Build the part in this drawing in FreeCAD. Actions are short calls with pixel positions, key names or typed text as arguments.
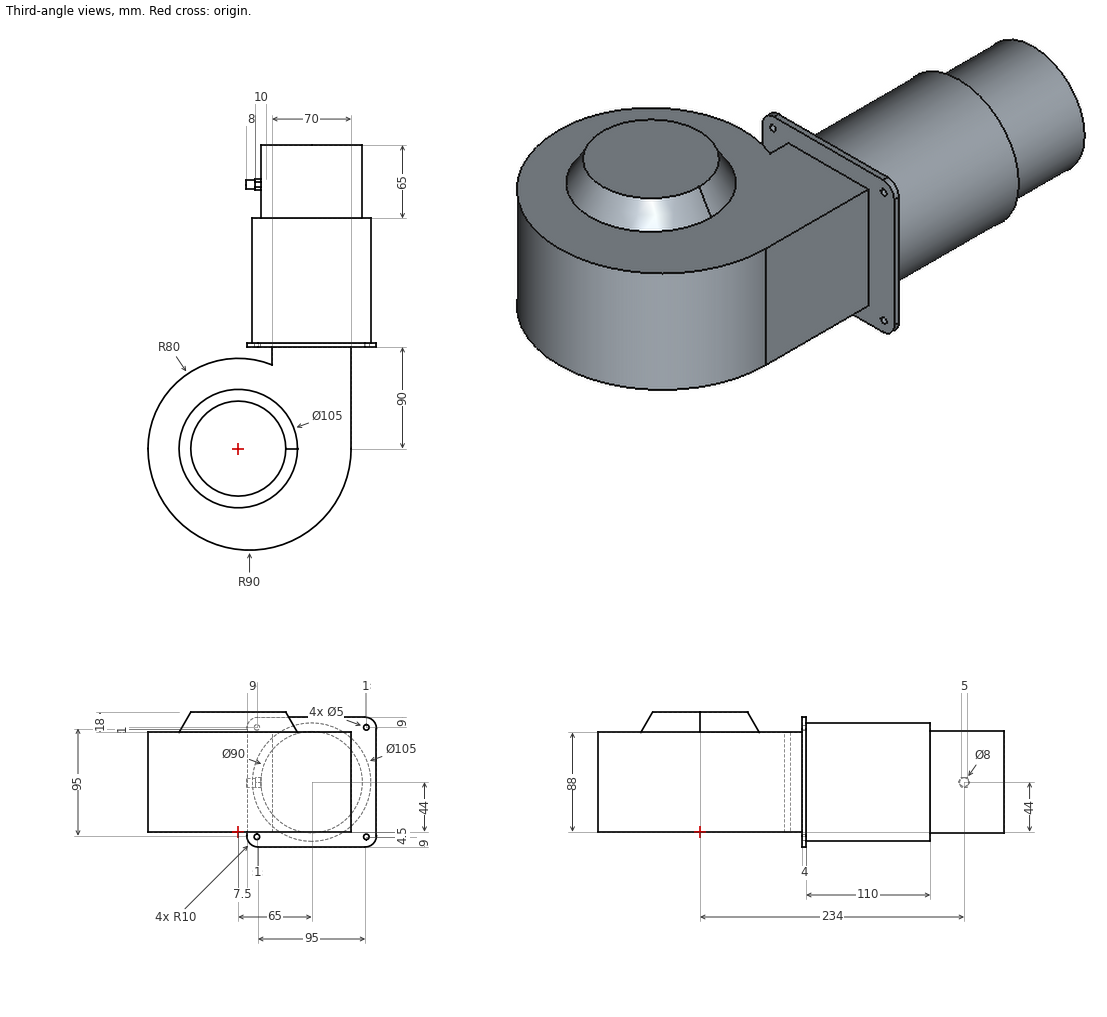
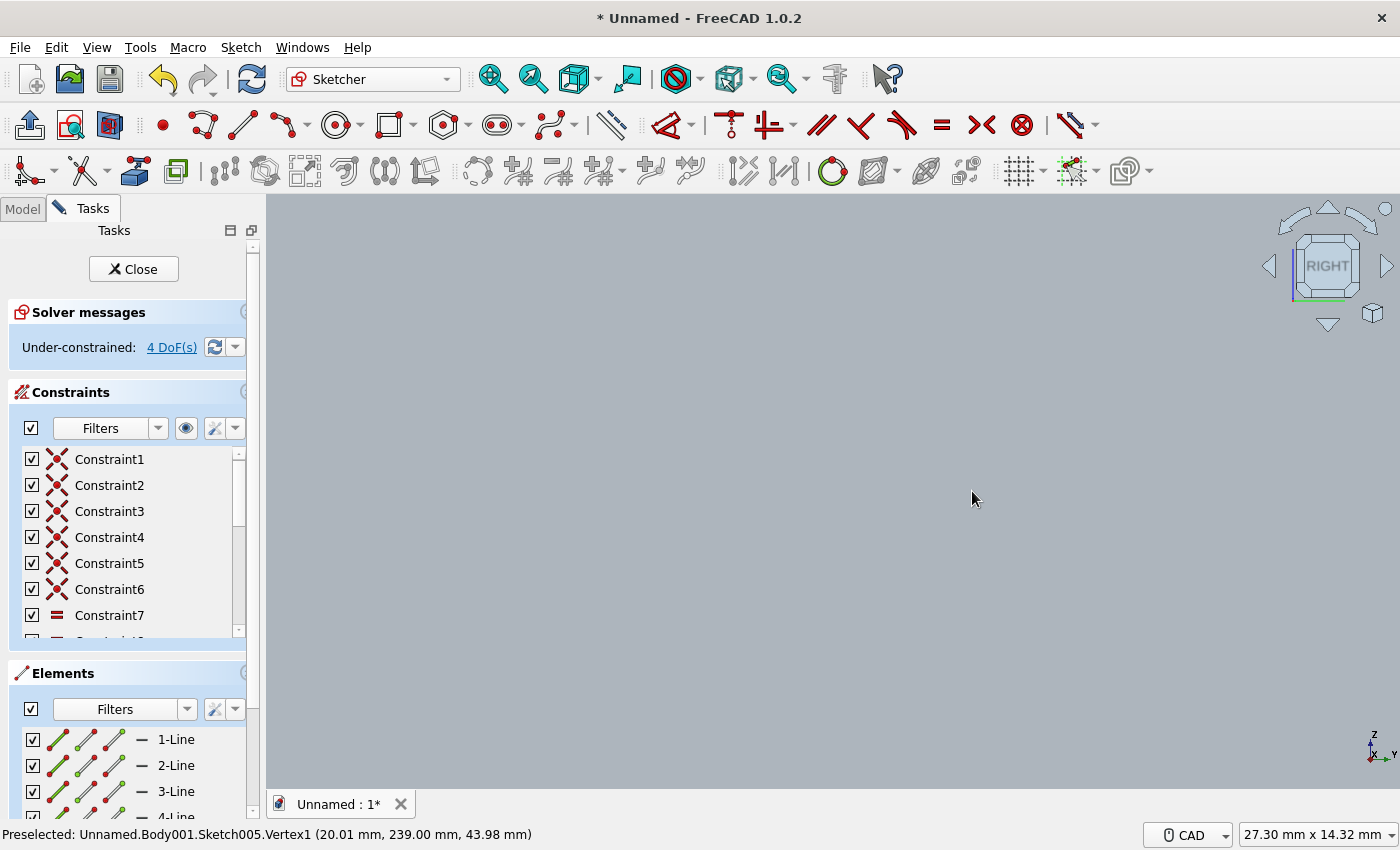
click(806, 312)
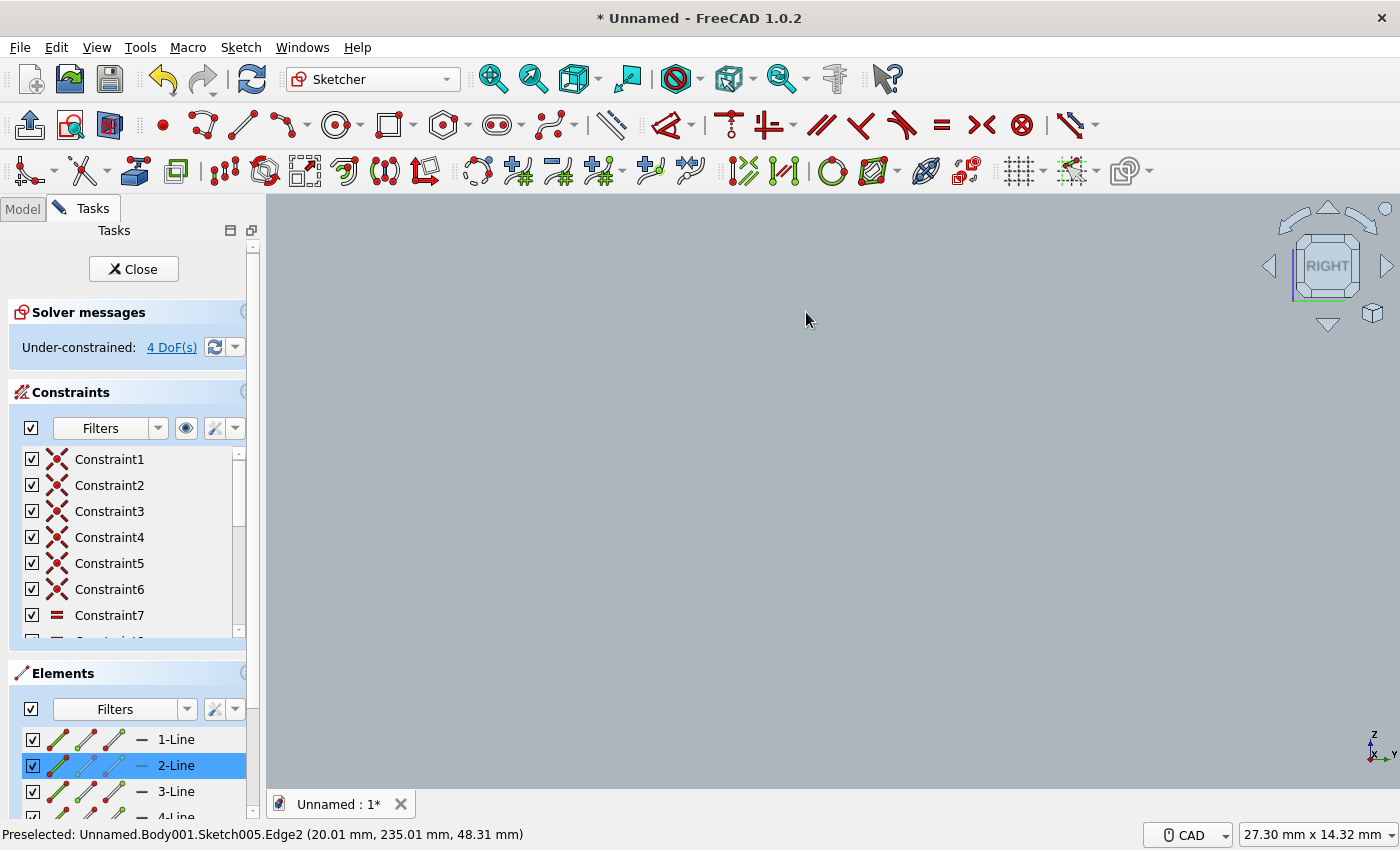
key(h)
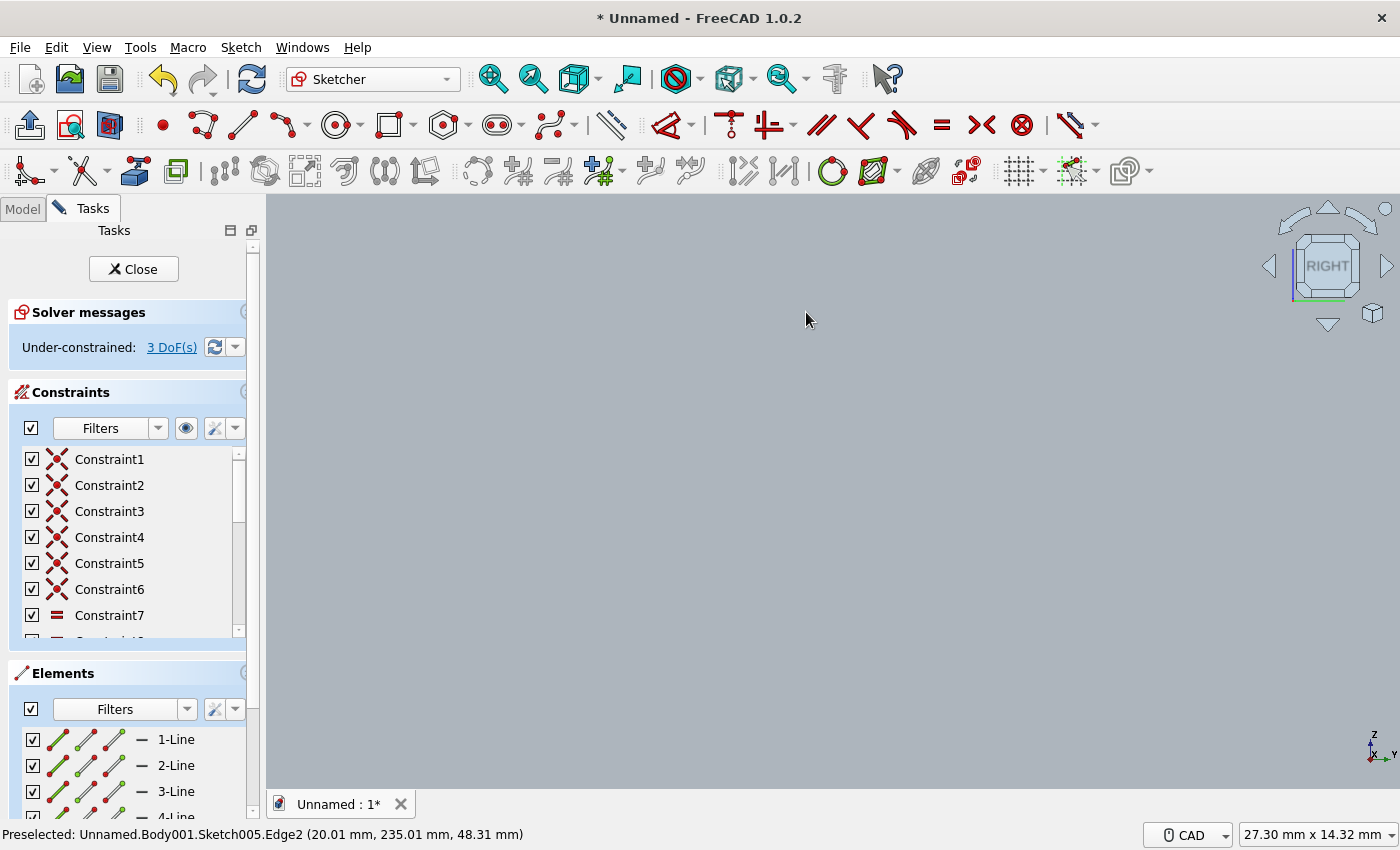
click(666, 126)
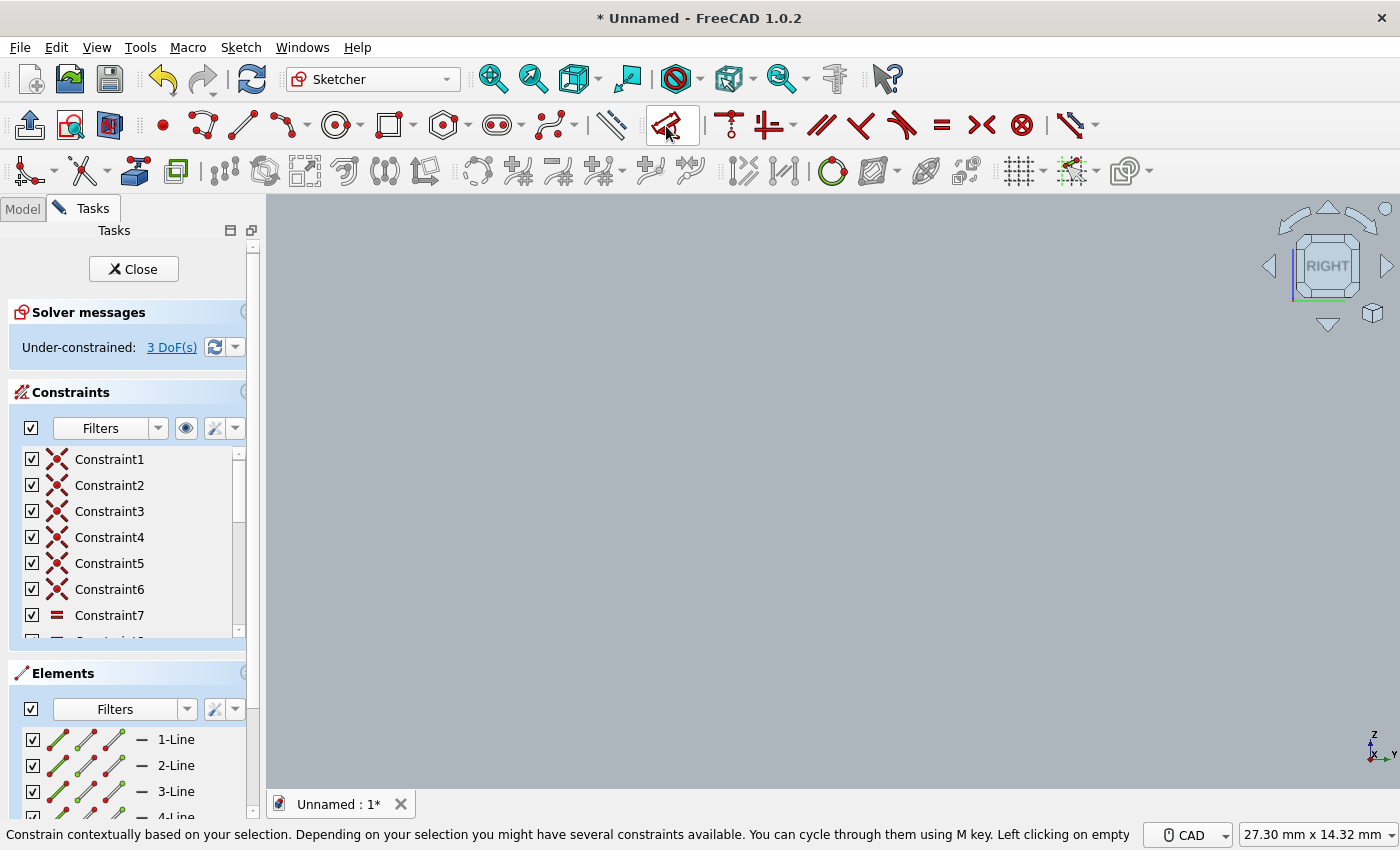
click(806, 312)
click(691, 278)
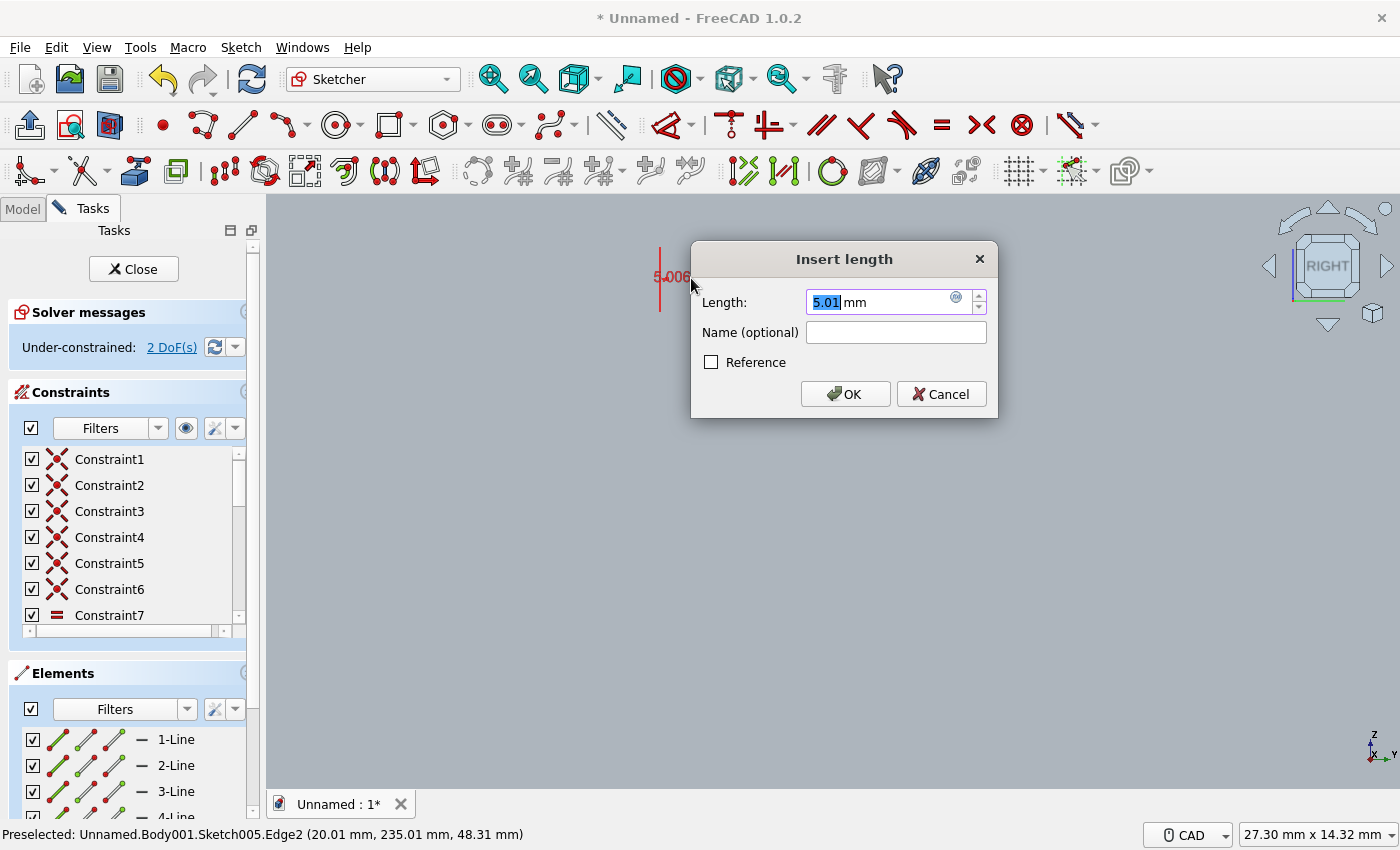
text(5)
key(Return)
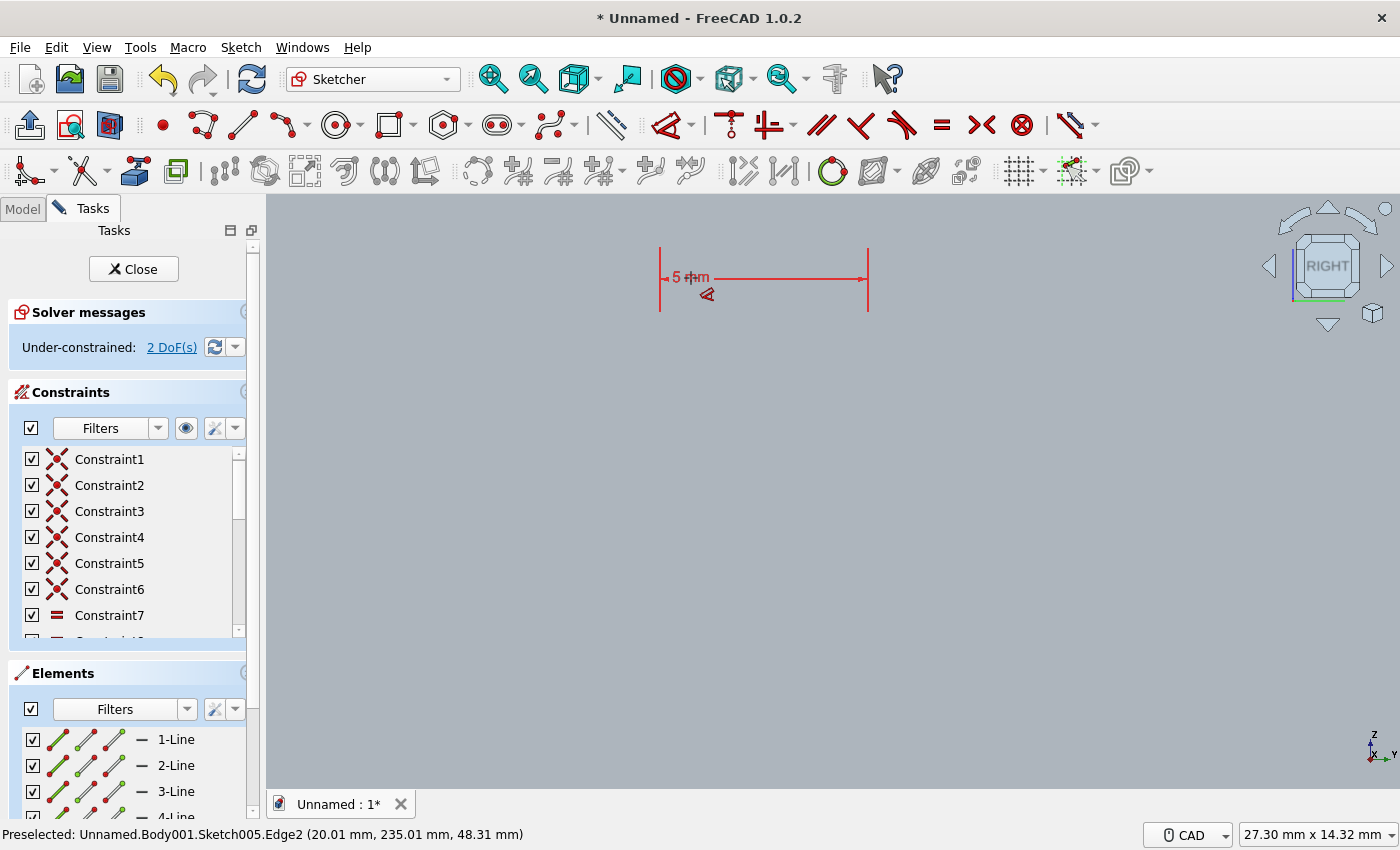
click(764, 492)
click(798, 627)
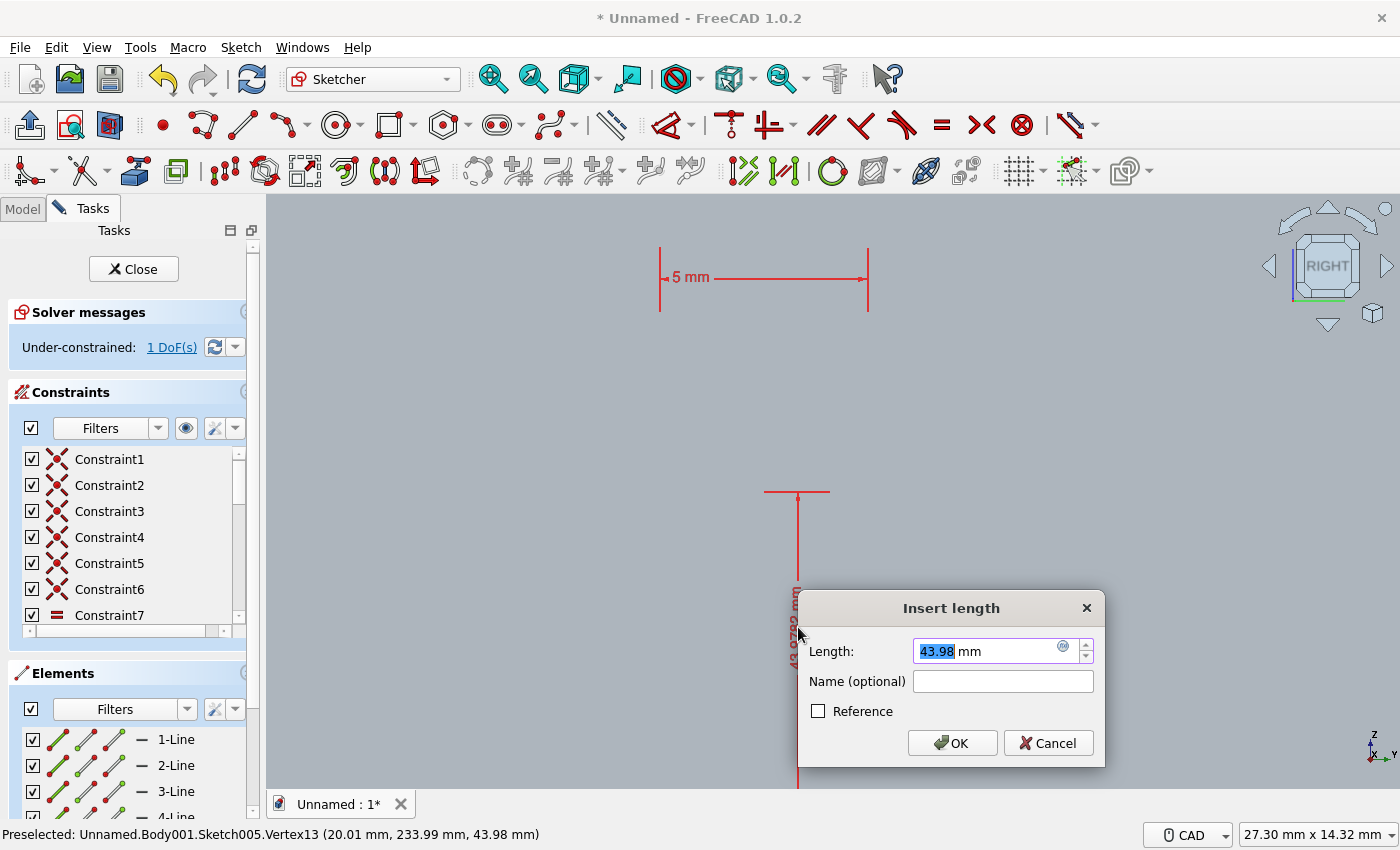
text(44)
key(Return)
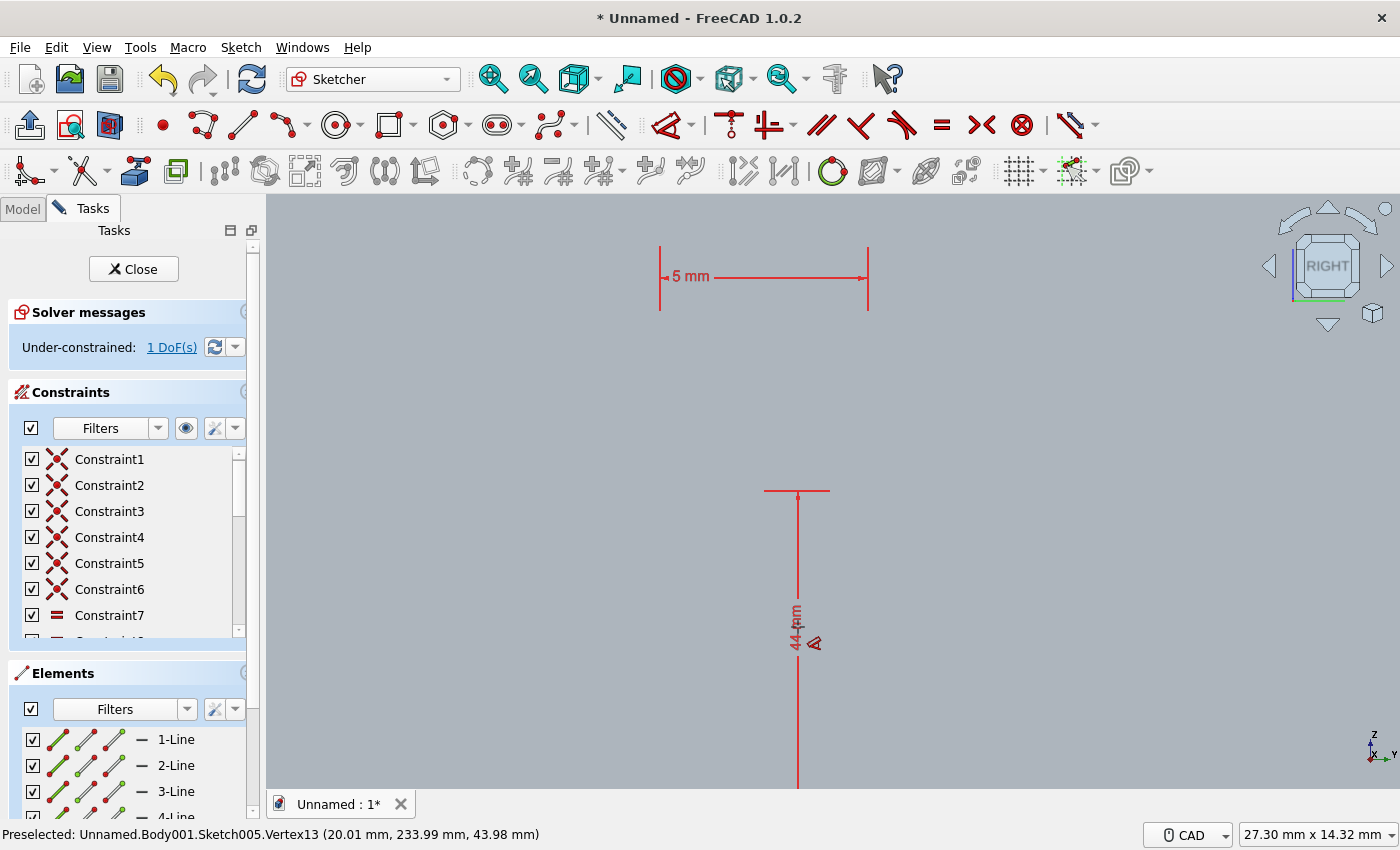
click(764, 491)
click(529, 457)